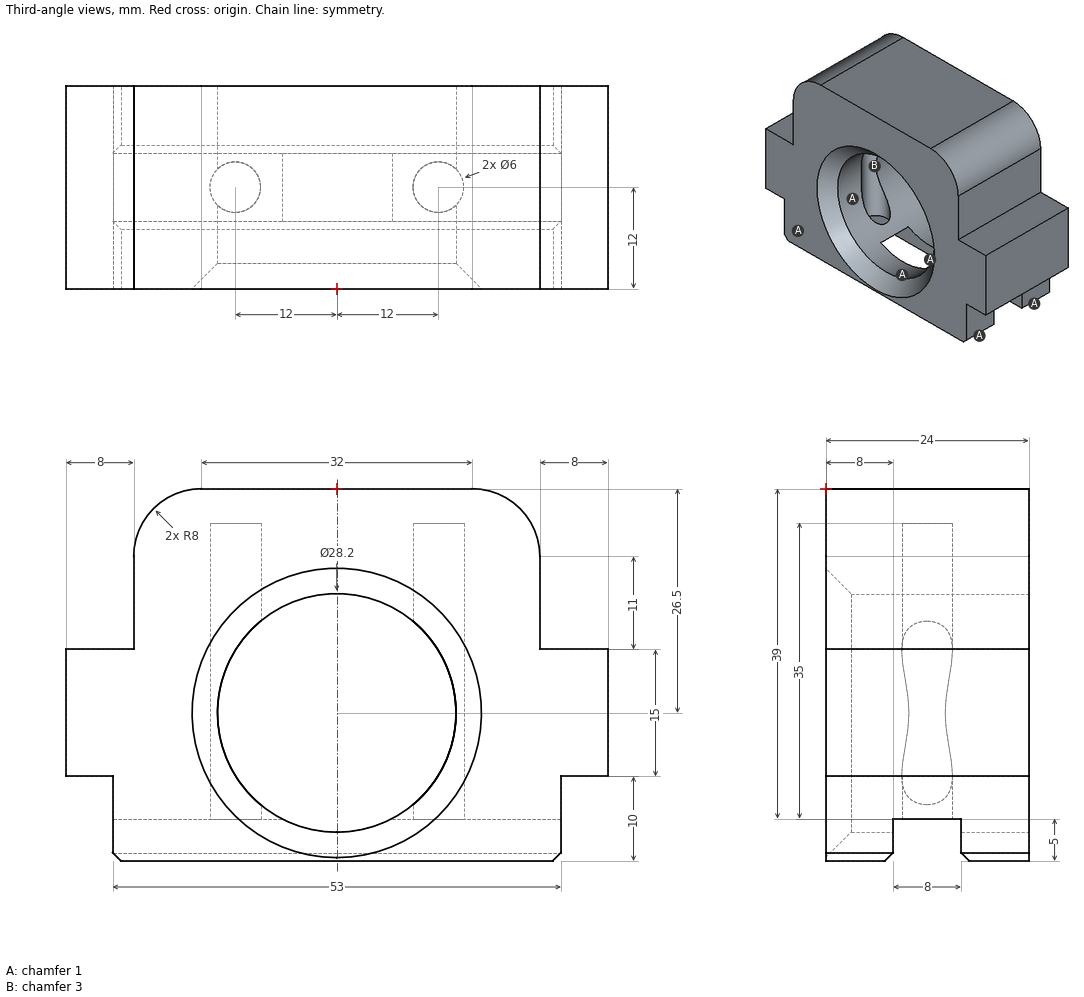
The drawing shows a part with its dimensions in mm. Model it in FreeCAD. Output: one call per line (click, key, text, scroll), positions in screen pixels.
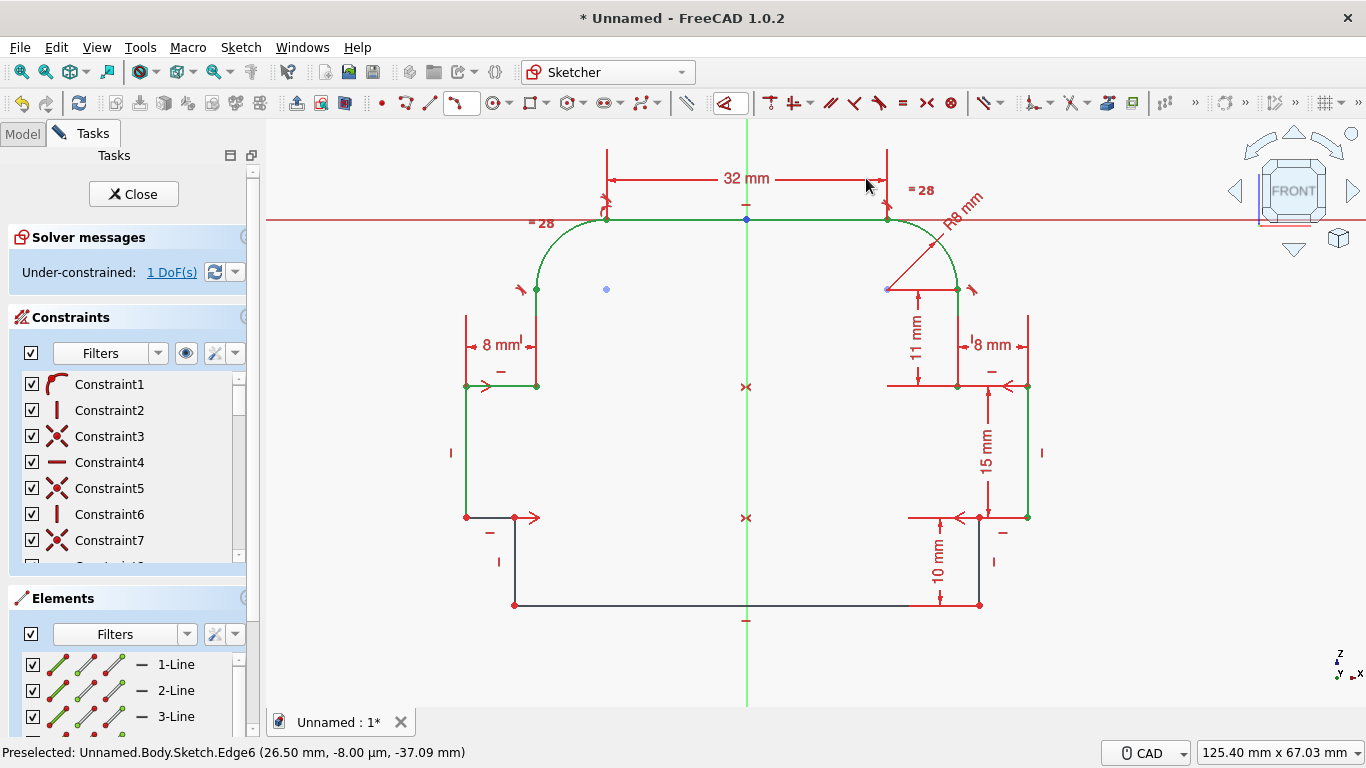
click(840, 606)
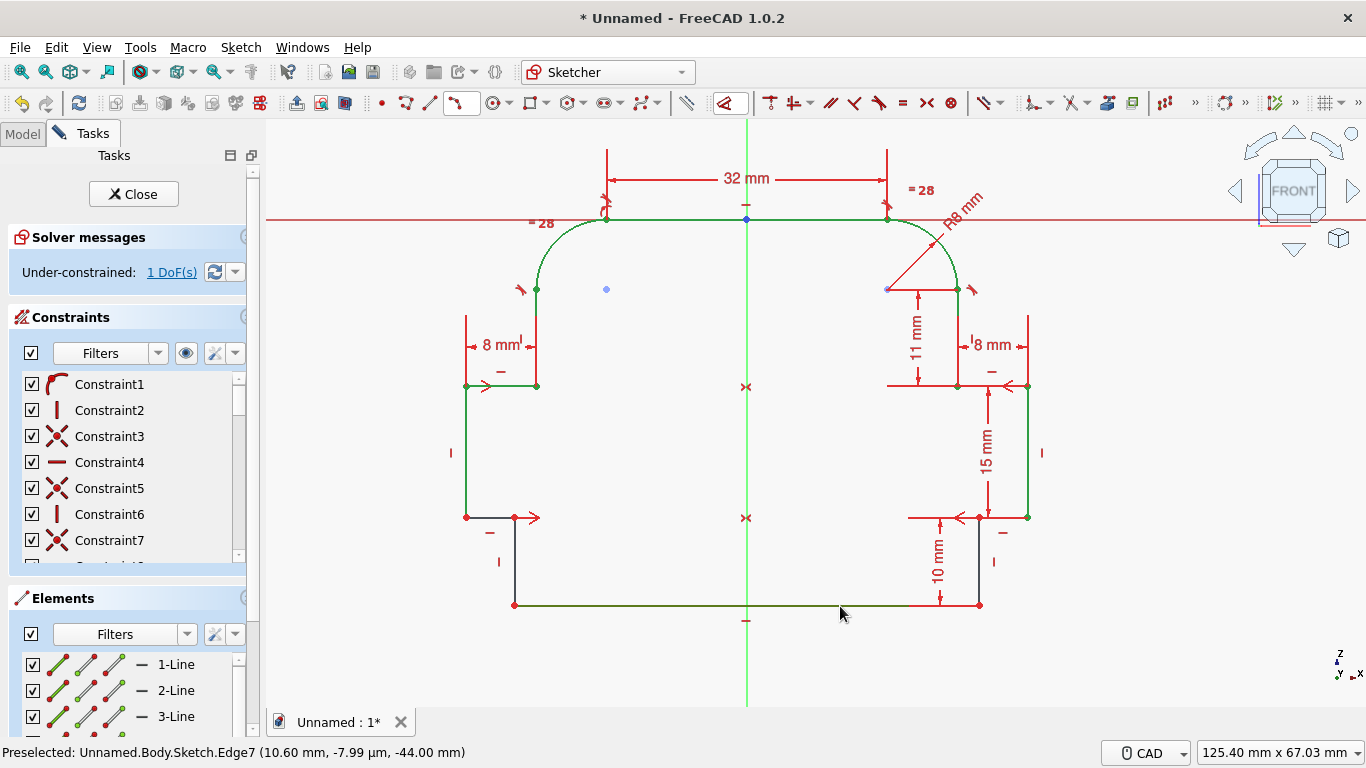
key(l)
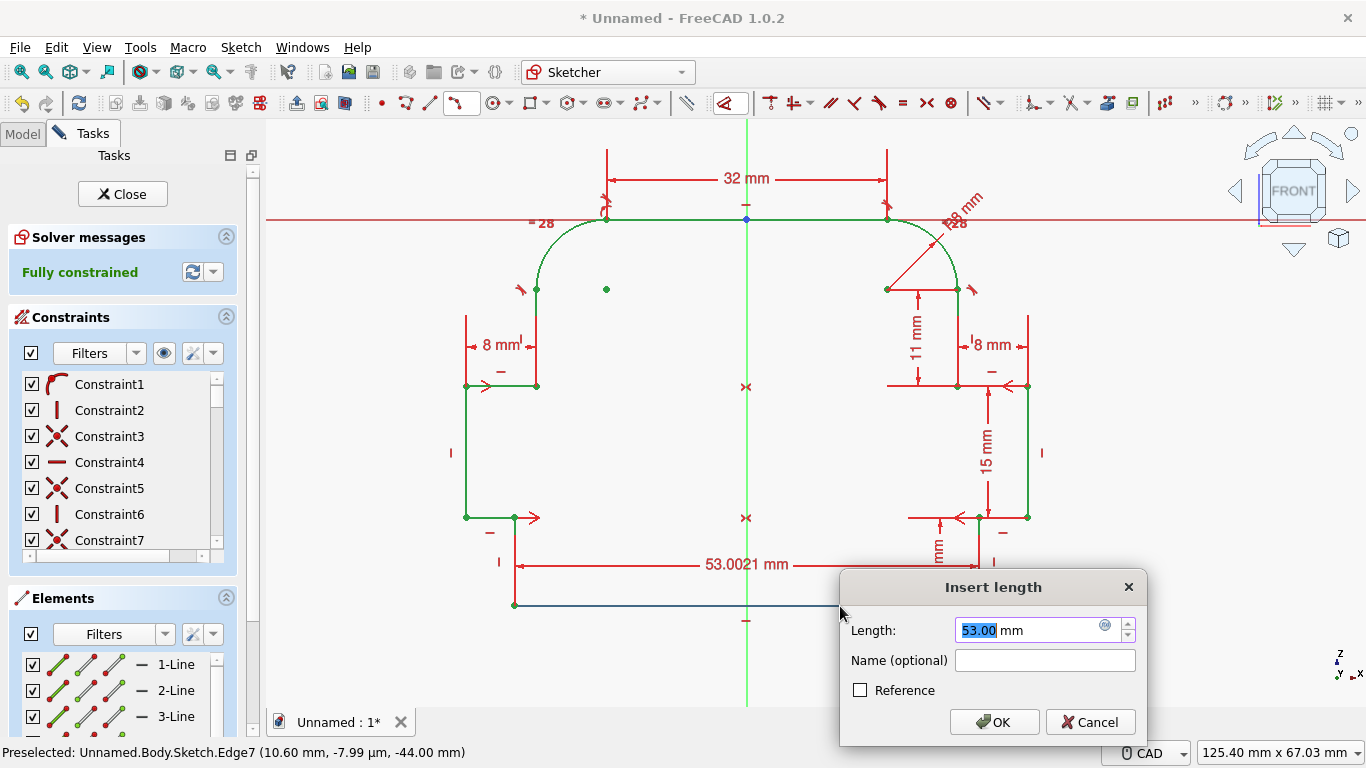
text(53)
key(Return)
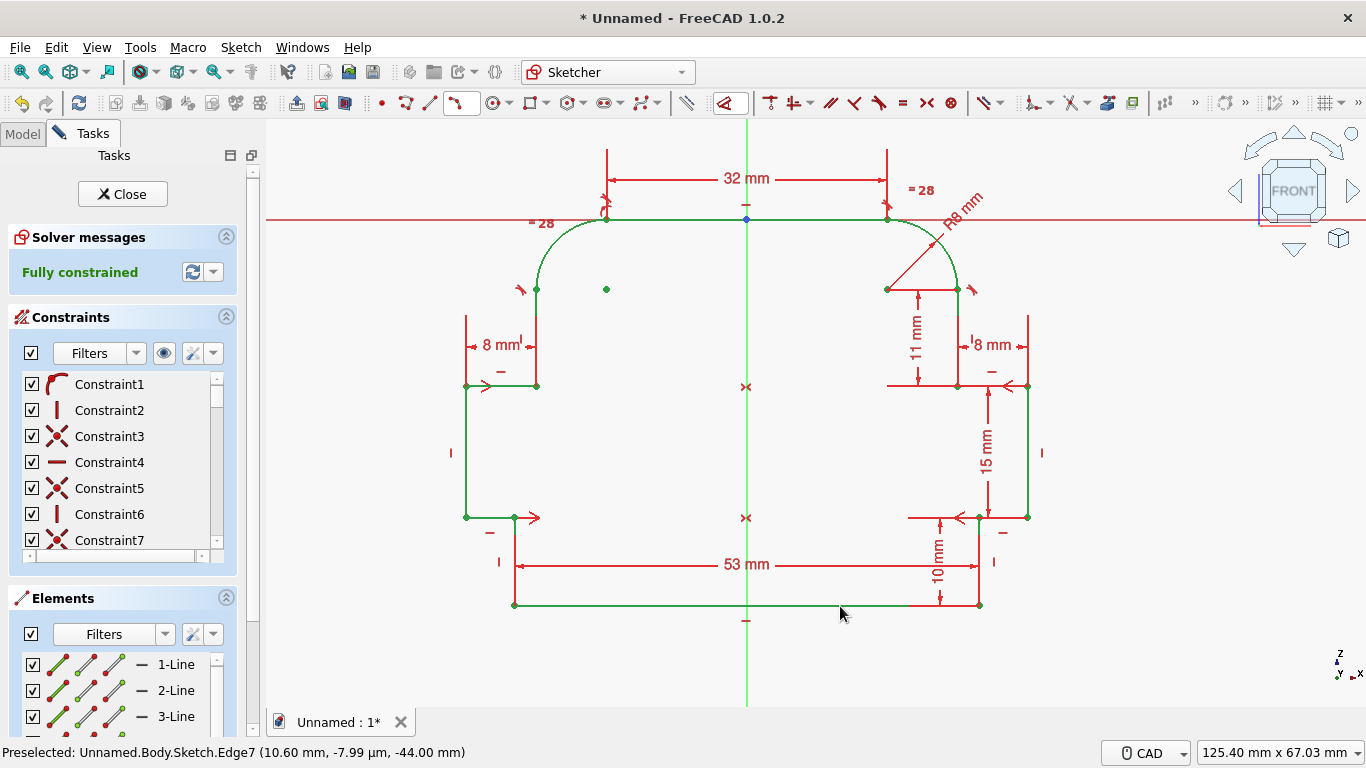
click(123, 194)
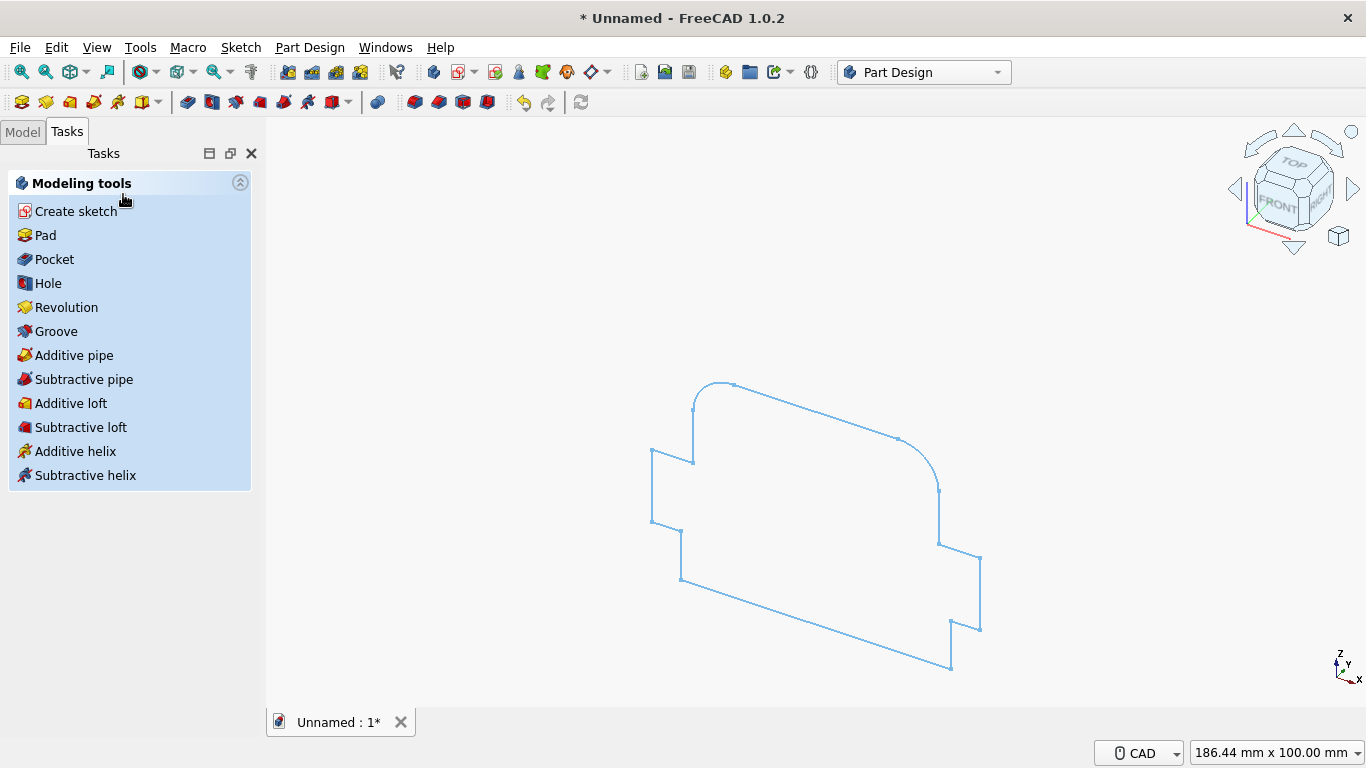
click(22, 102)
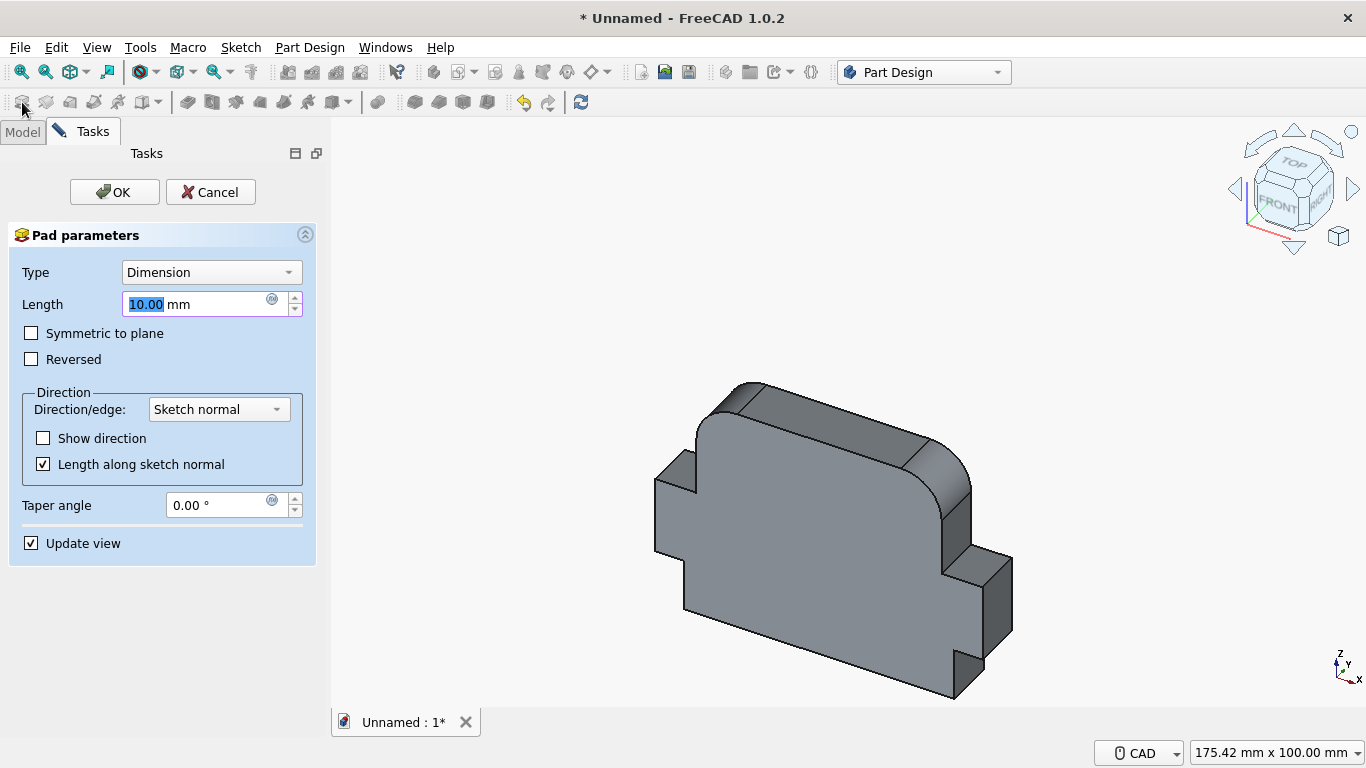
text(24)
key(Tab)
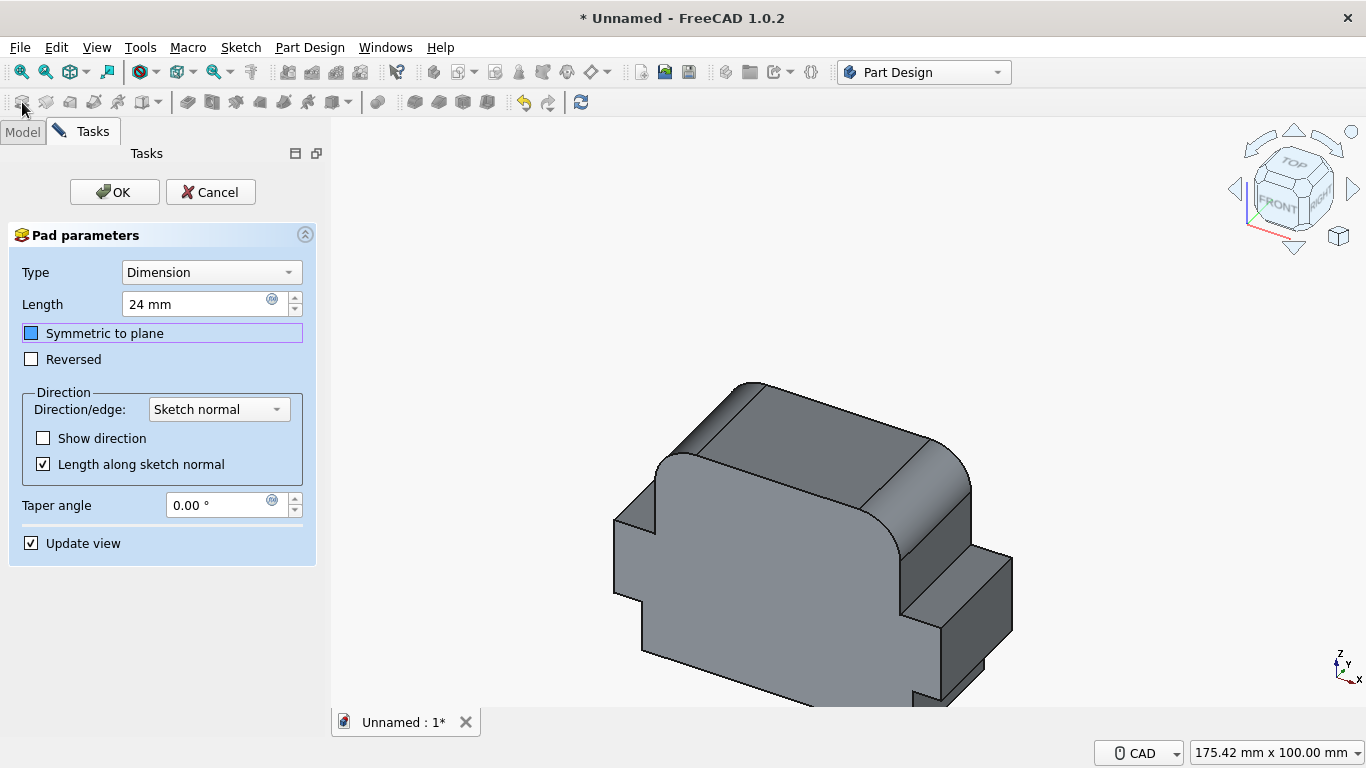
click(30, 359)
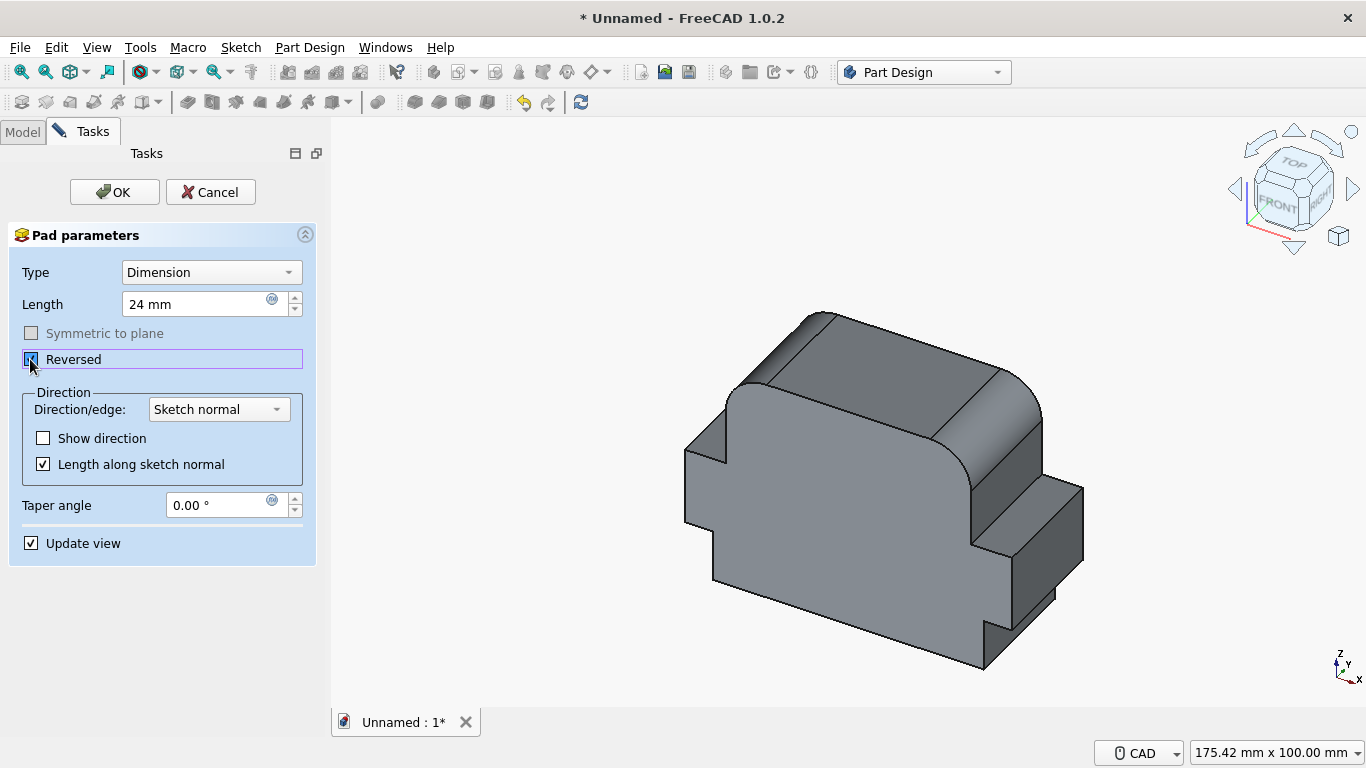
click(115, 192)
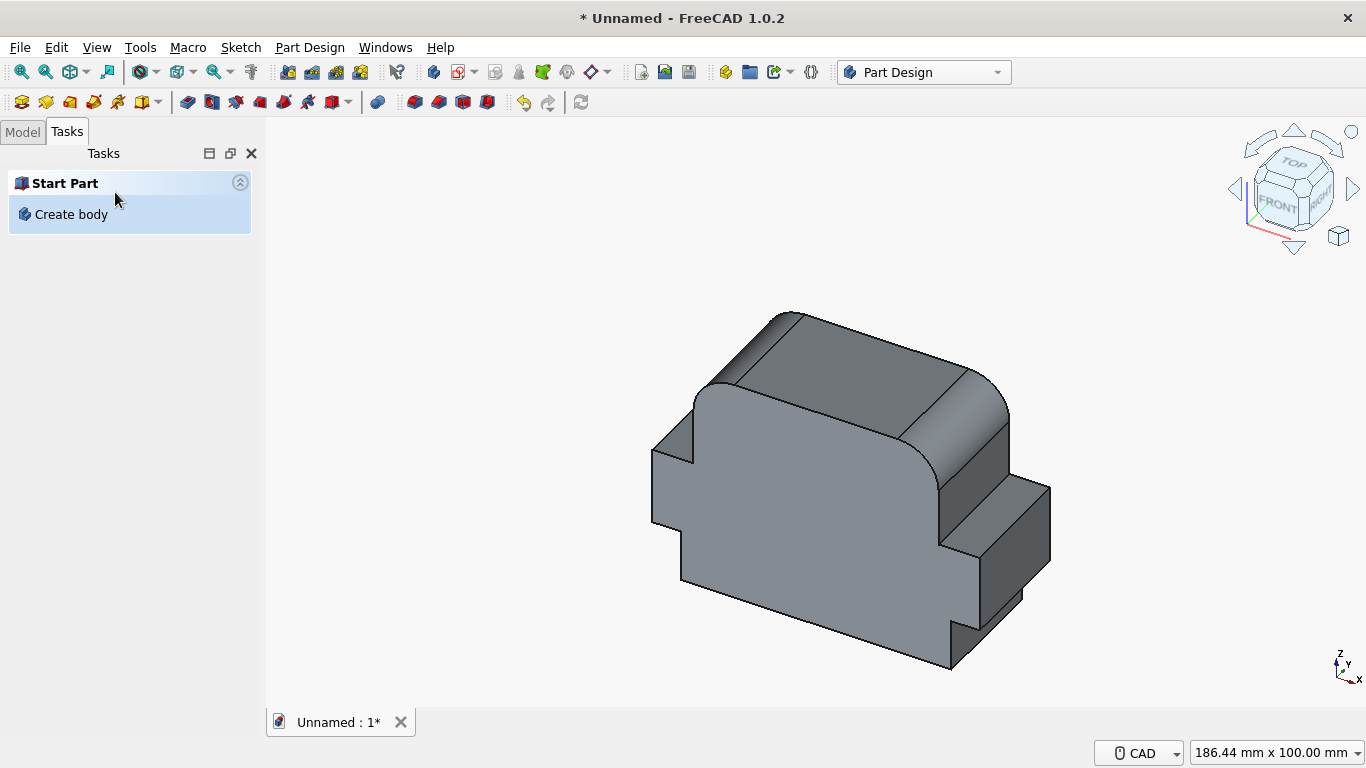
key(6)